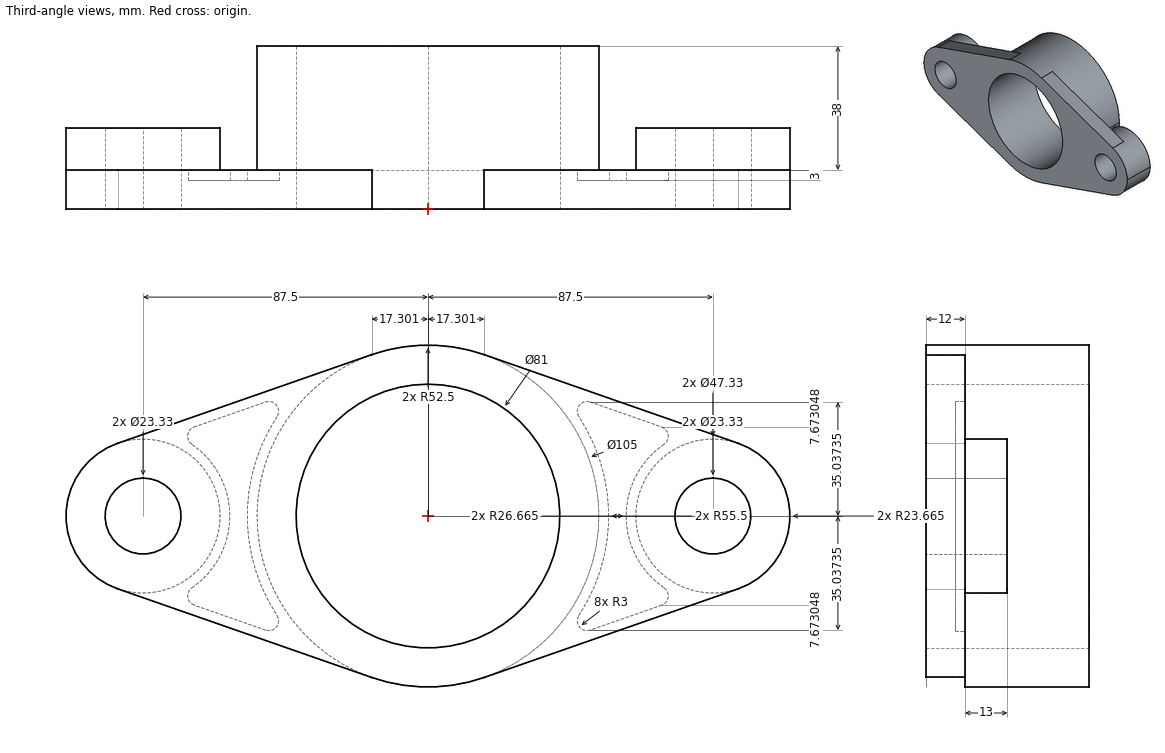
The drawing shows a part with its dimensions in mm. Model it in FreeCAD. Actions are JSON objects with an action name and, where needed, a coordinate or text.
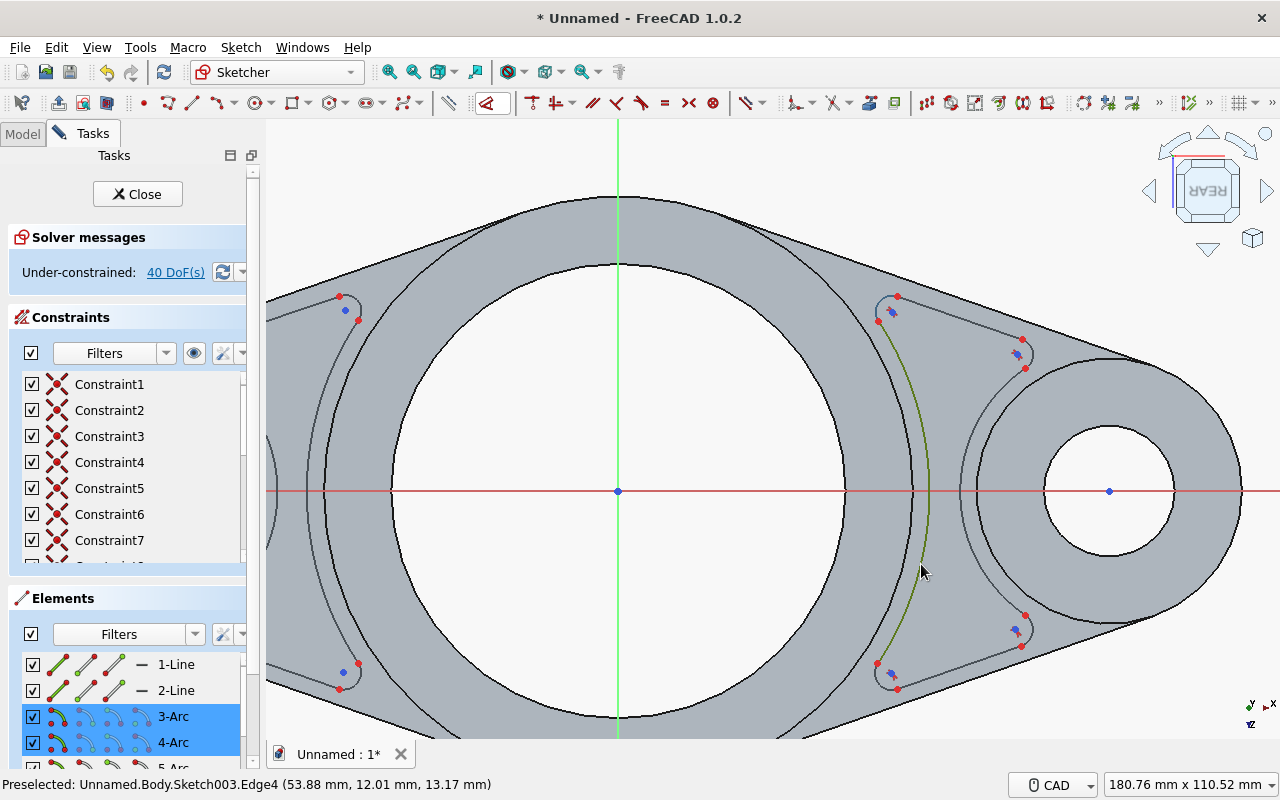
{"action": "left_click", "coordinate": [642, 104]}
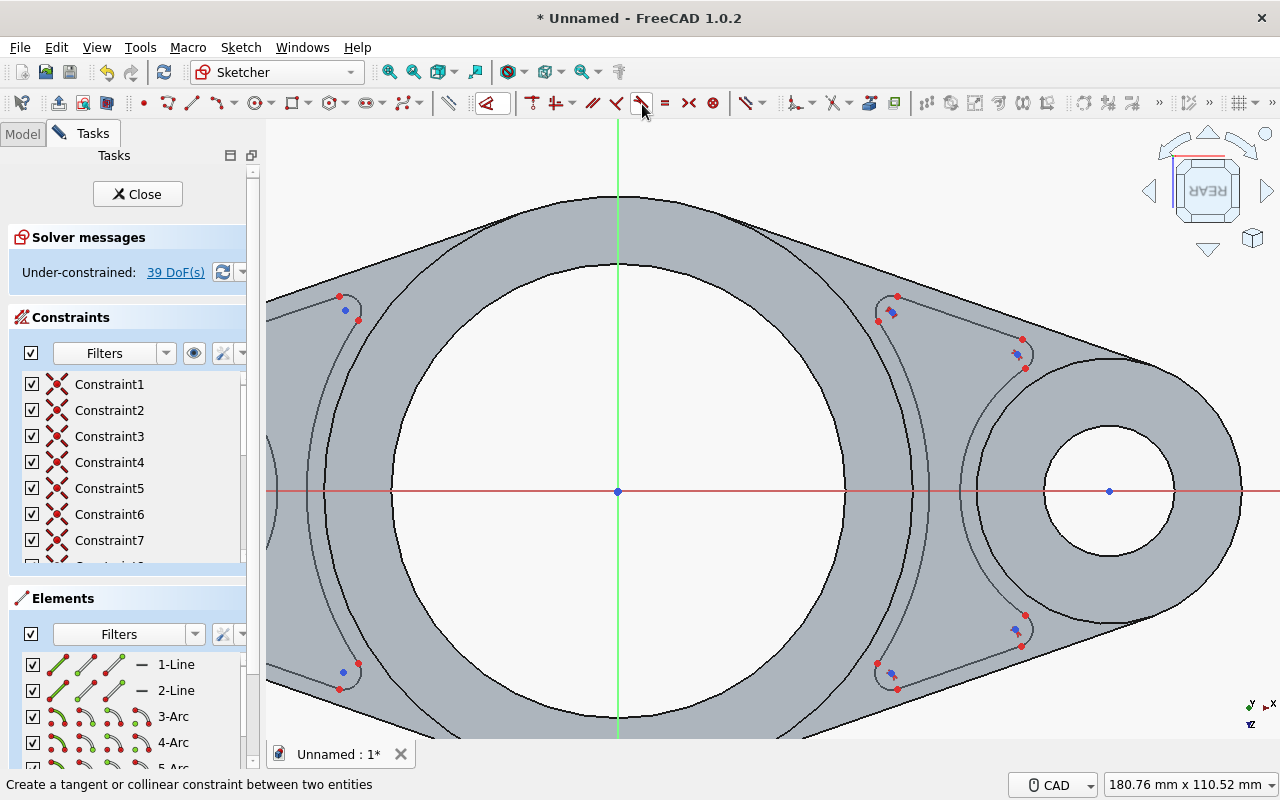
{"action": "left_click", "coordinate": [921, 564]}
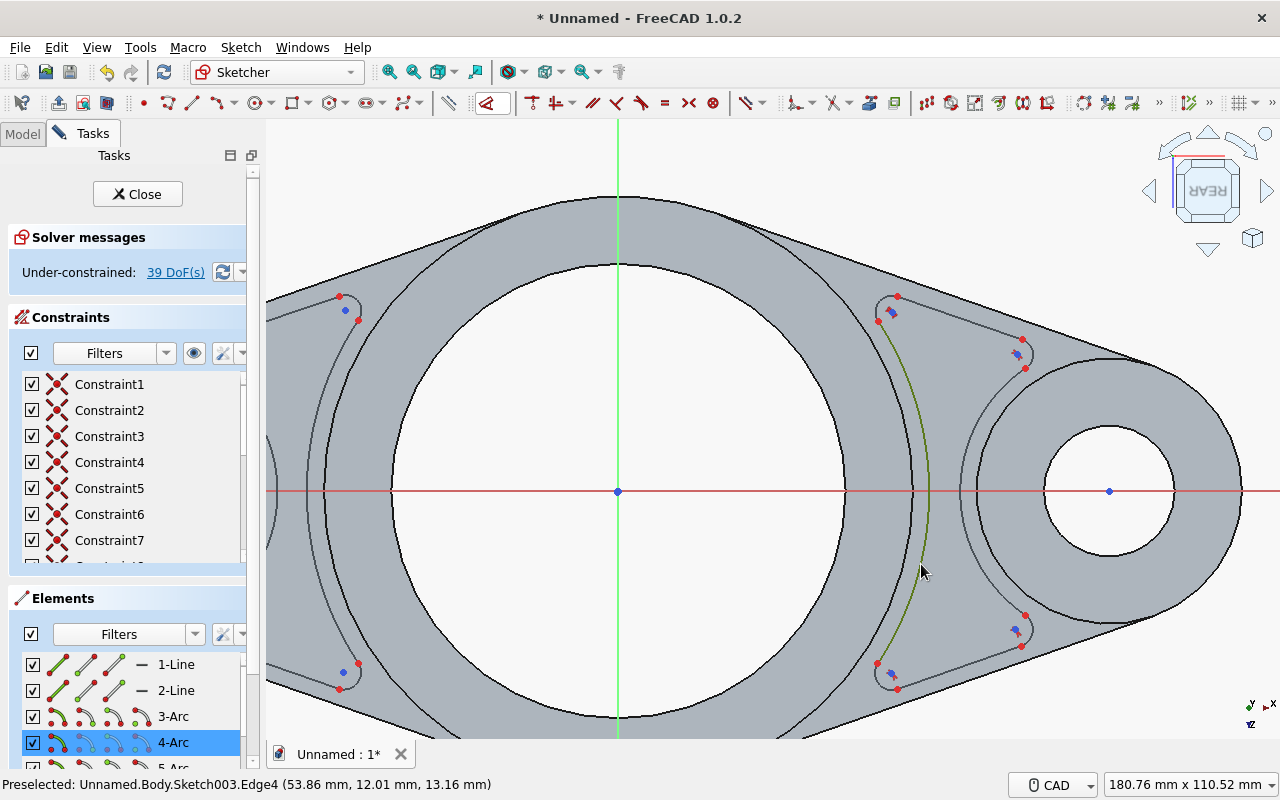
{"action": "left_click", "coordinate": [875, 676]}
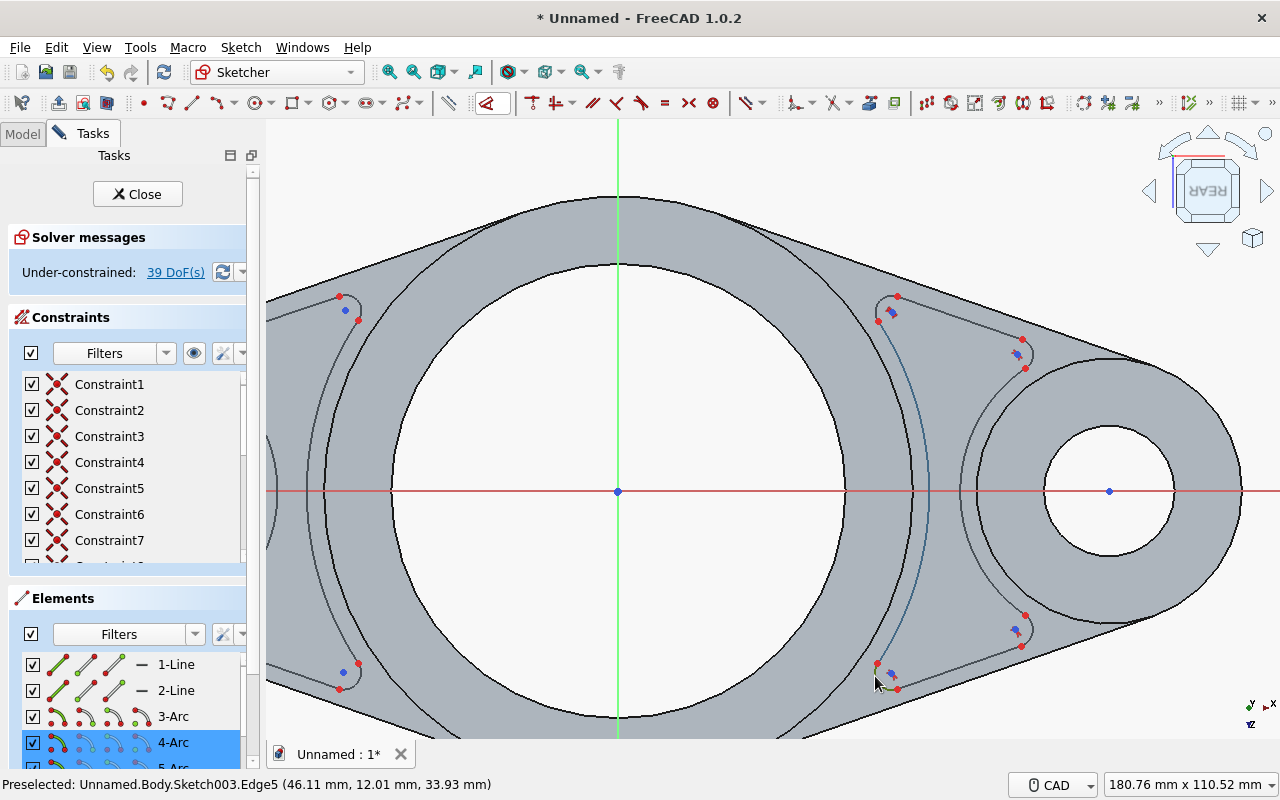
{"action": "left_click", "coordinate": [642, 104]}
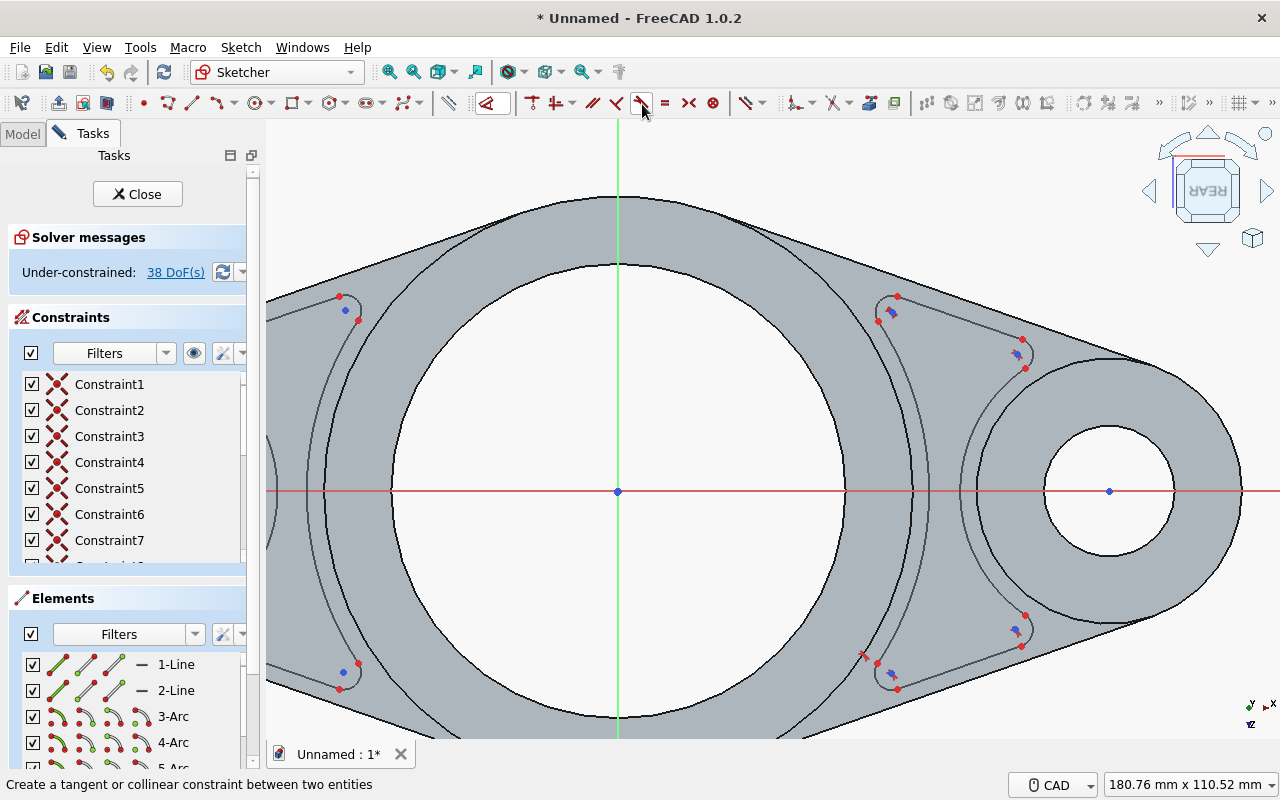
{"action": "left_click", "coordinate": [1030, 639]}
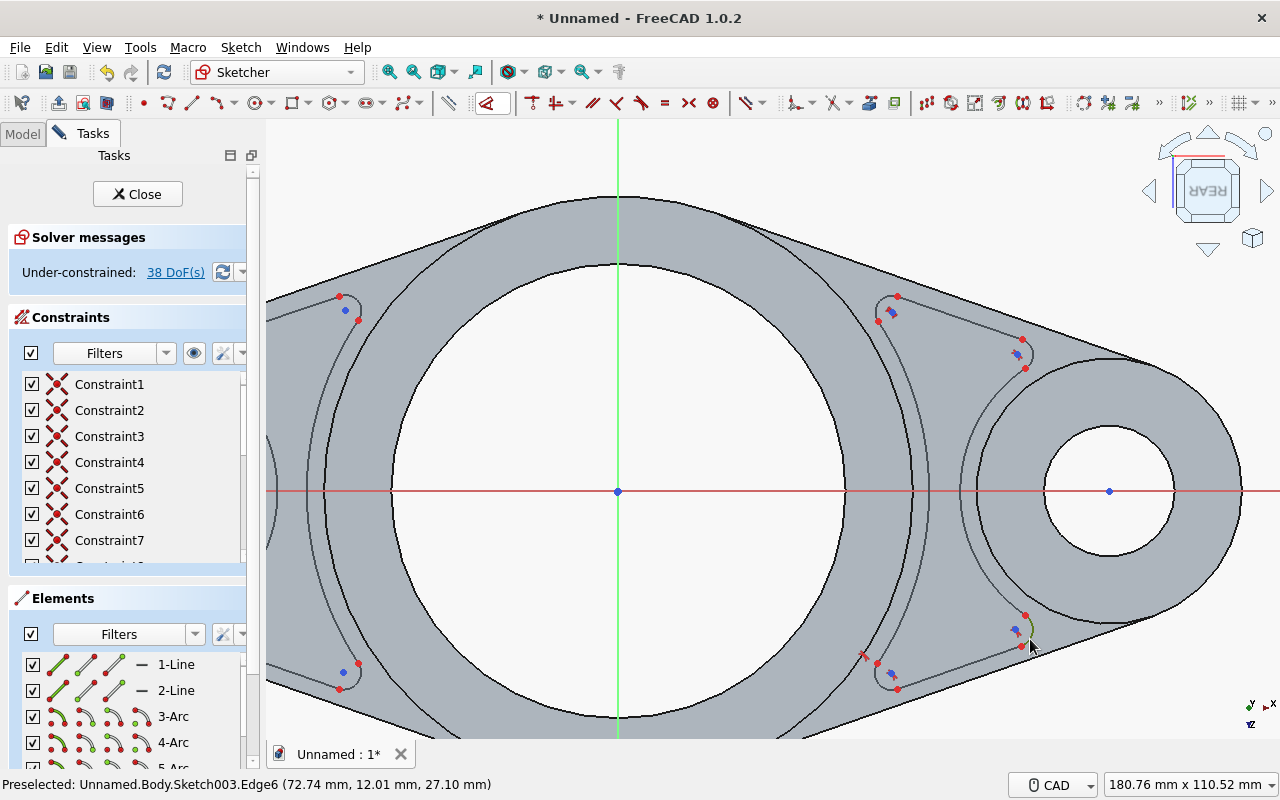
{"action": "left_click", "coordinate": [971, 435]}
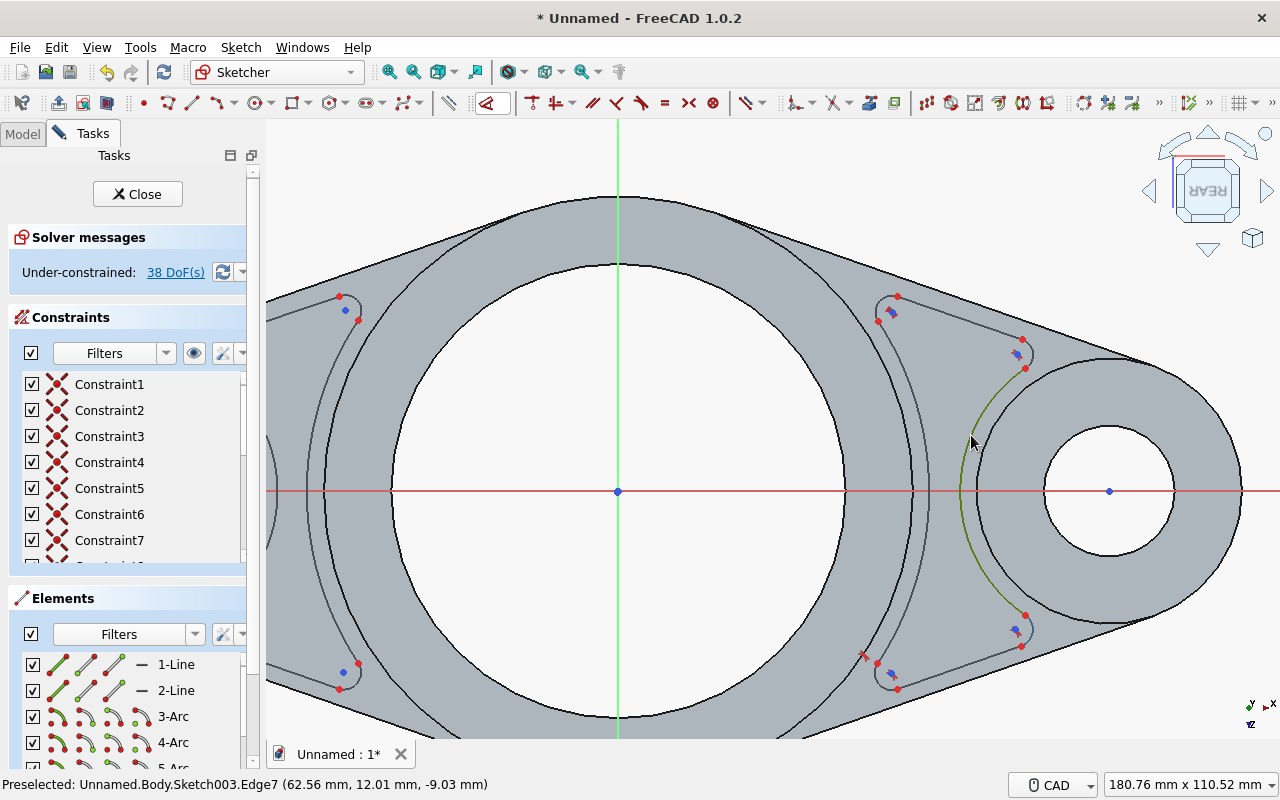
{"action": "left_click", "coordinate": [642, 104]}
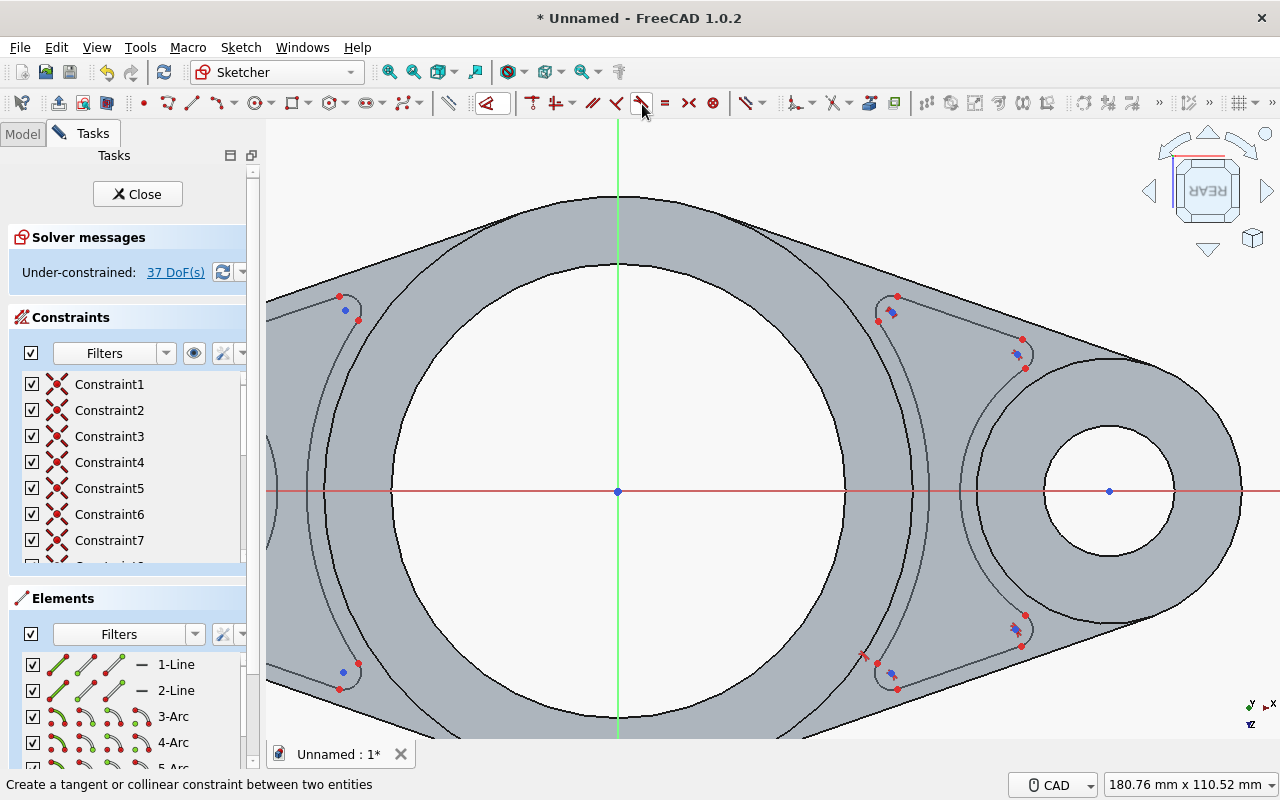
{"action": "left_click", "coordinate": [971, 435]}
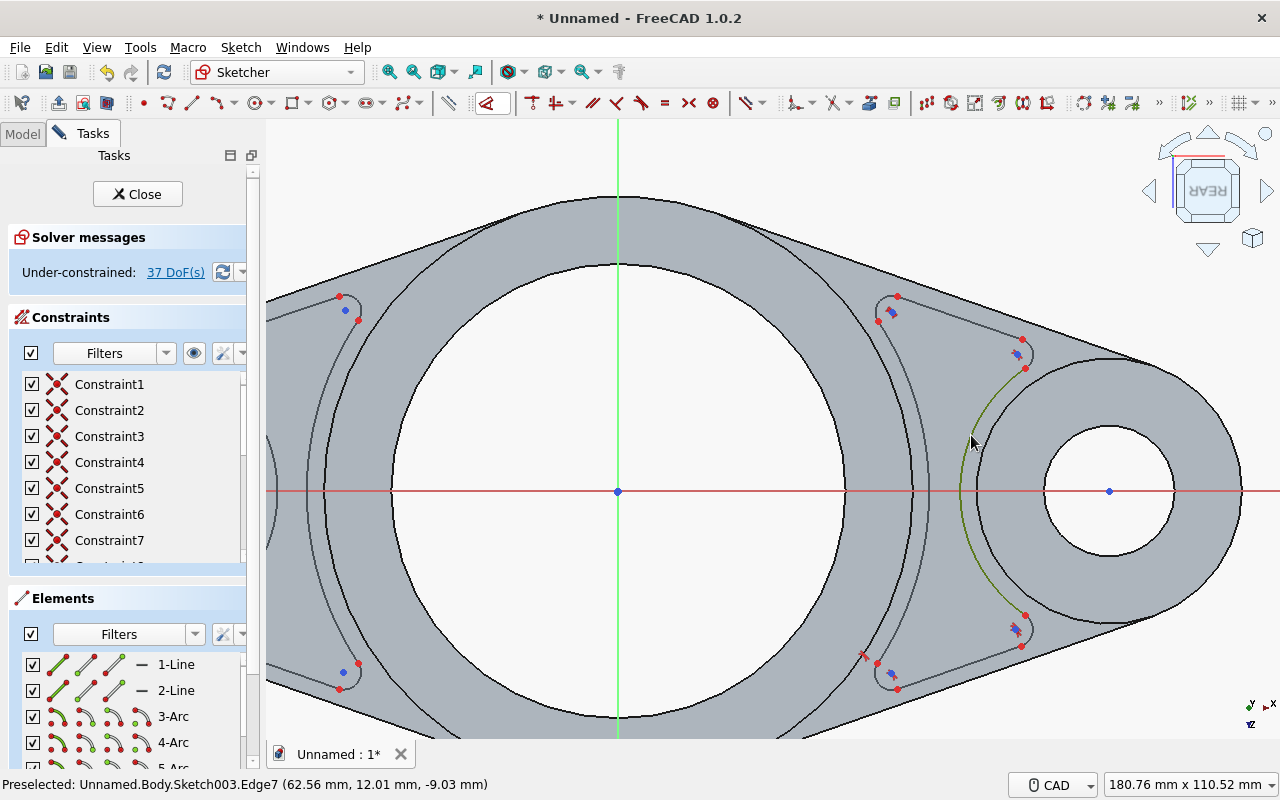
{"action": "scroll", "coordinate": [1032, 360], "scroll_direction": "up", "scroll_amount": 2}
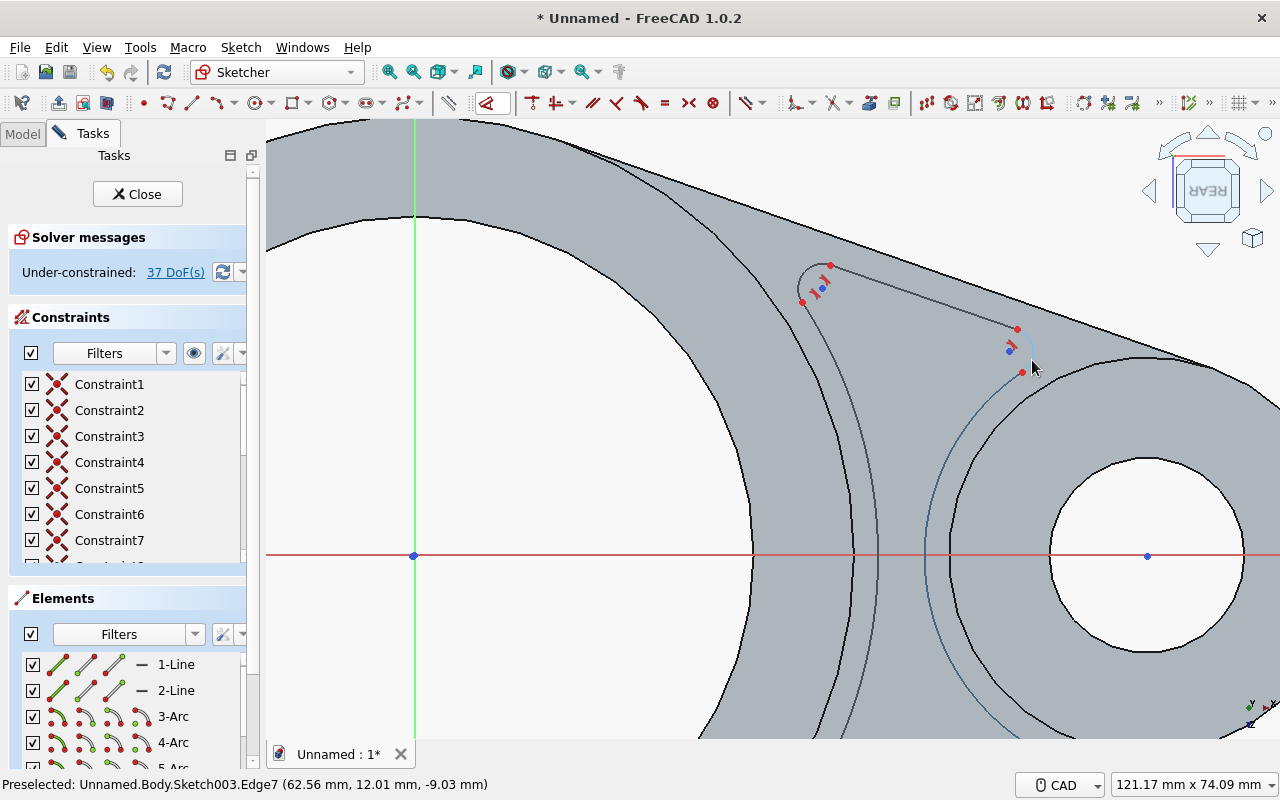
{"action": "left_click", "coordinate": [1032, 360]}